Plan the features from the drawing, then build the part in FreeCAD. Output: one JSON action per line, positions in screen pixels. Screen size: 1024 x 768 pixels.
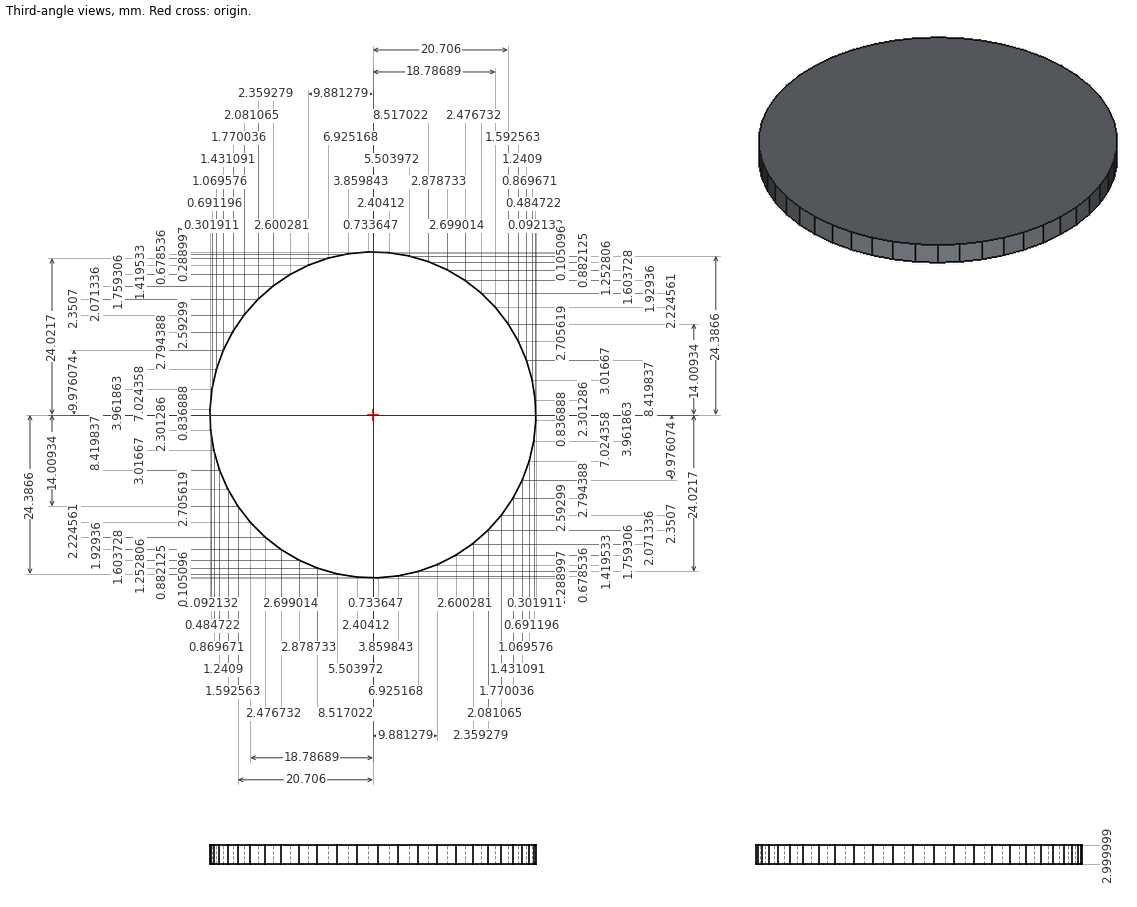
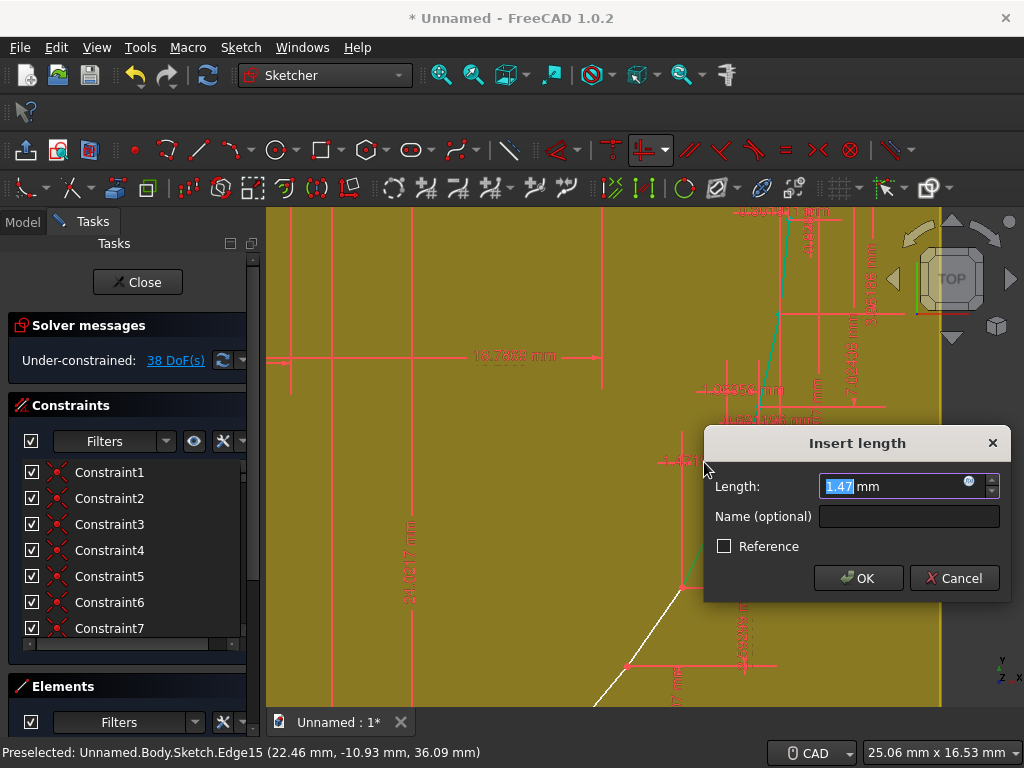
{"action": "type", "text": "1.431091"}
{"action": "key", "text": "Return"}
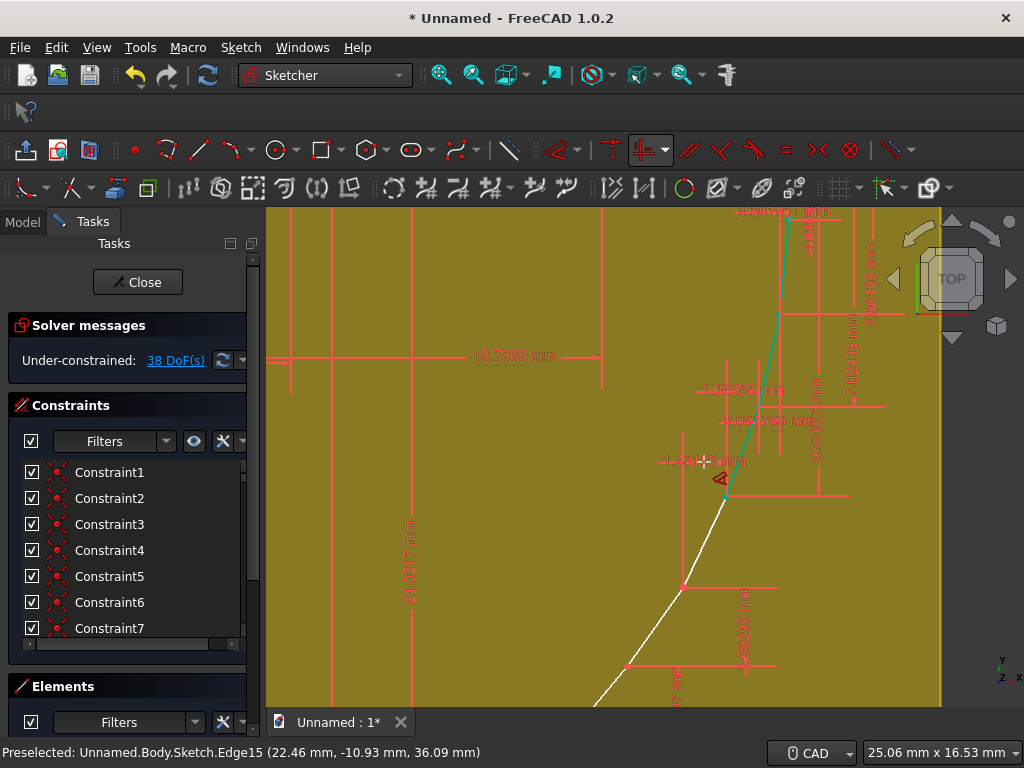
{"action": "left_click", "coordinate": [714, 524]}
{"action": "left_click", "coordinate": [761, 542]}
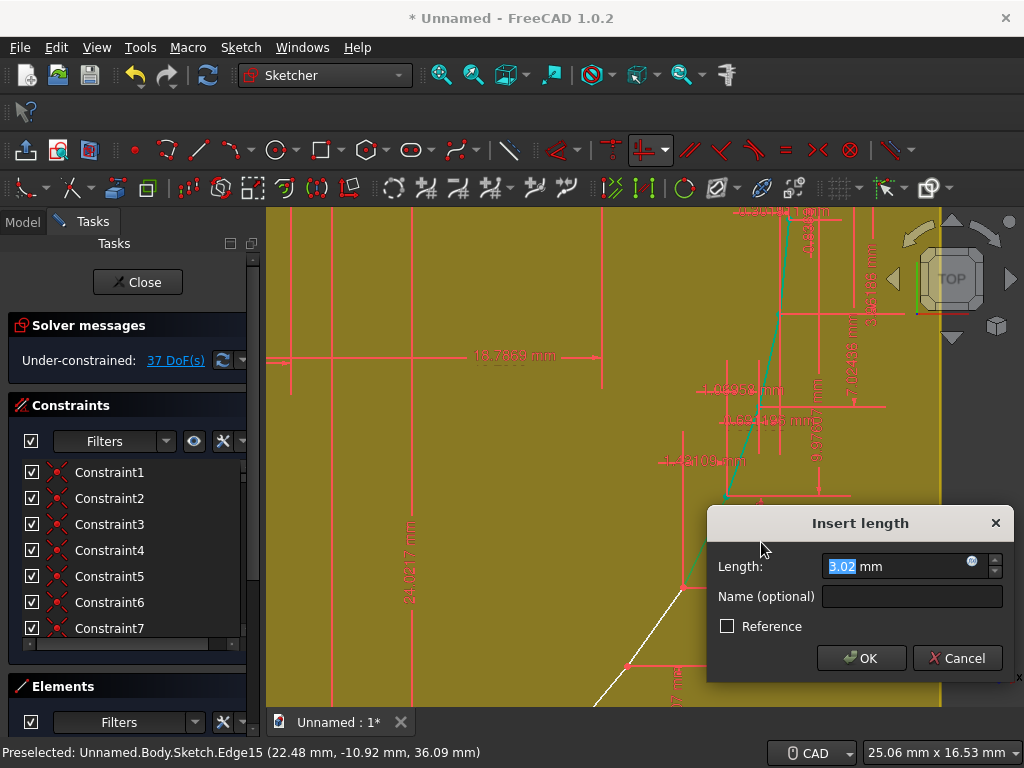
{"action": "type", "text": "2.794388"}
{"action": "key", "text": "Return"}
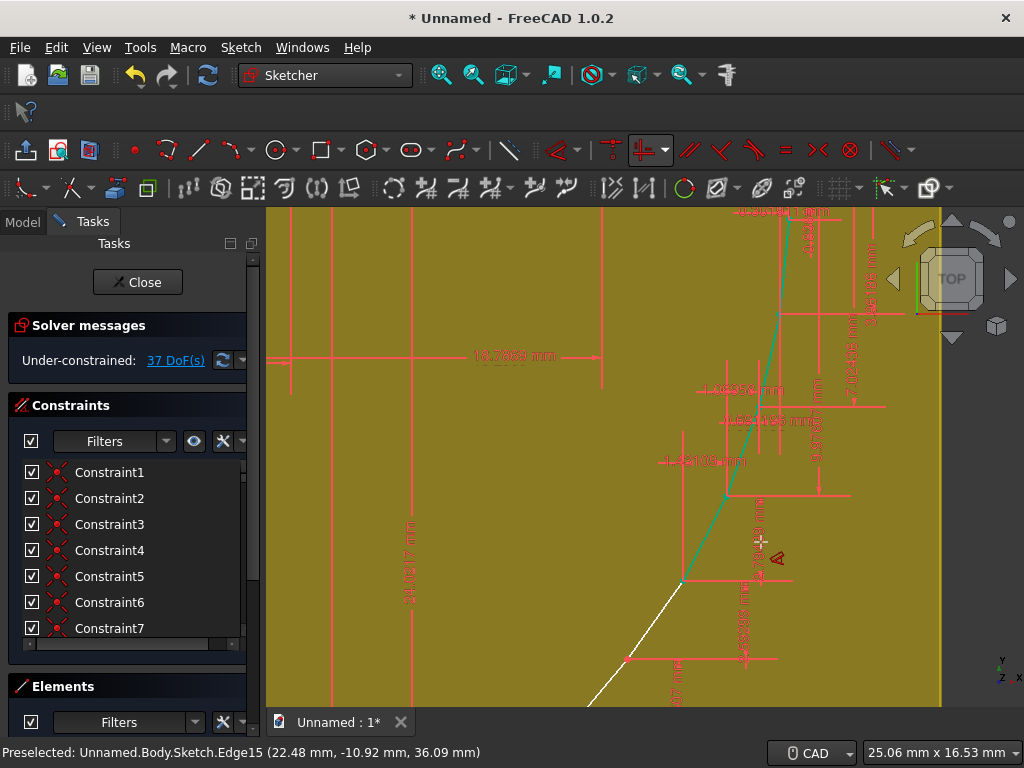
{"action": "left_click", "coordinate": [667, 604]}
{"action": "left_click", "coordinate": [656, 547]}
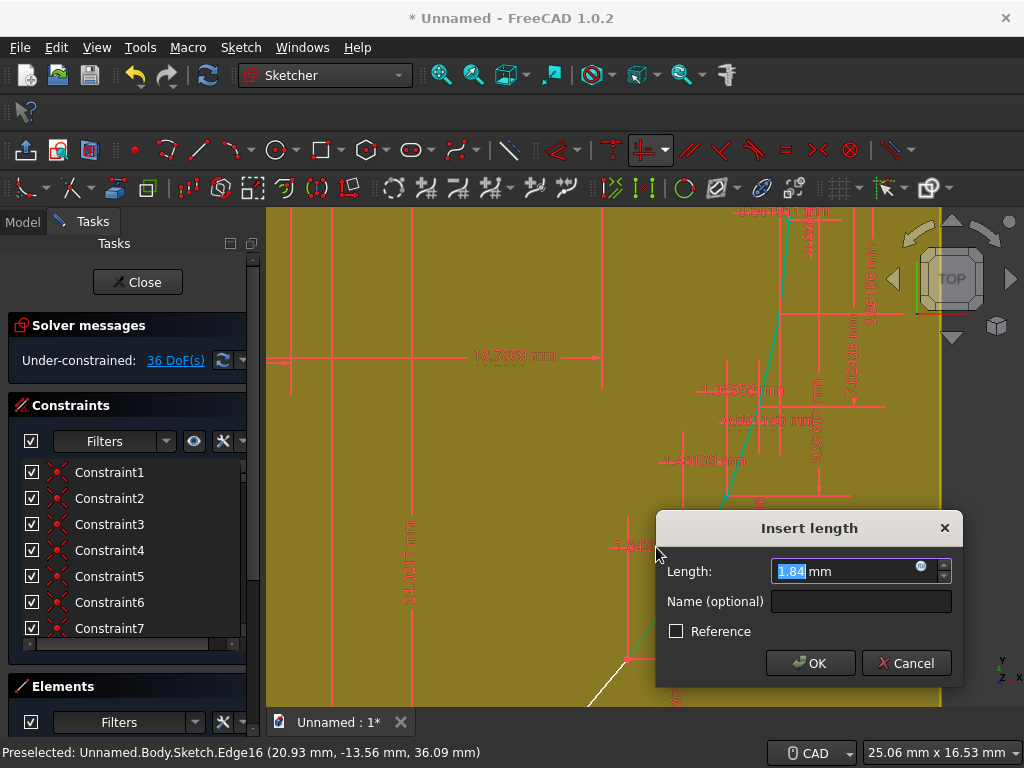
{"action": "type", "text": "1.770036"}
{"action": "key", "text": "Return"}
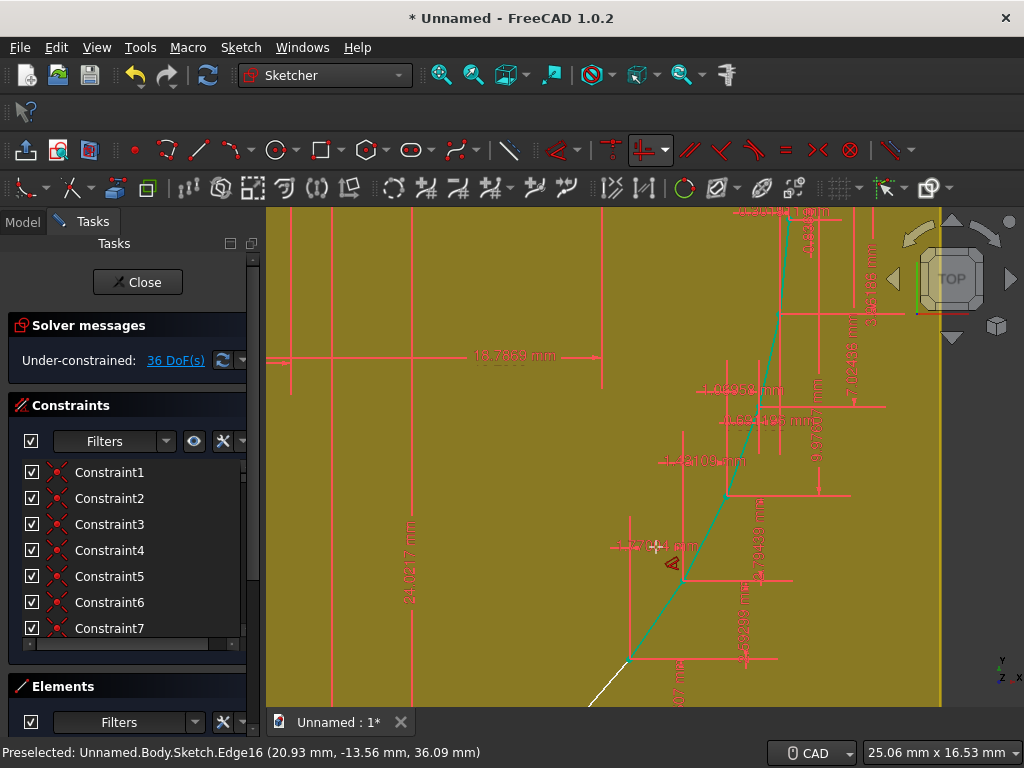
{"action": "left_click", "coordinate": [618, 673]}
{"action": "left_click", "coordinate": [599, 625]}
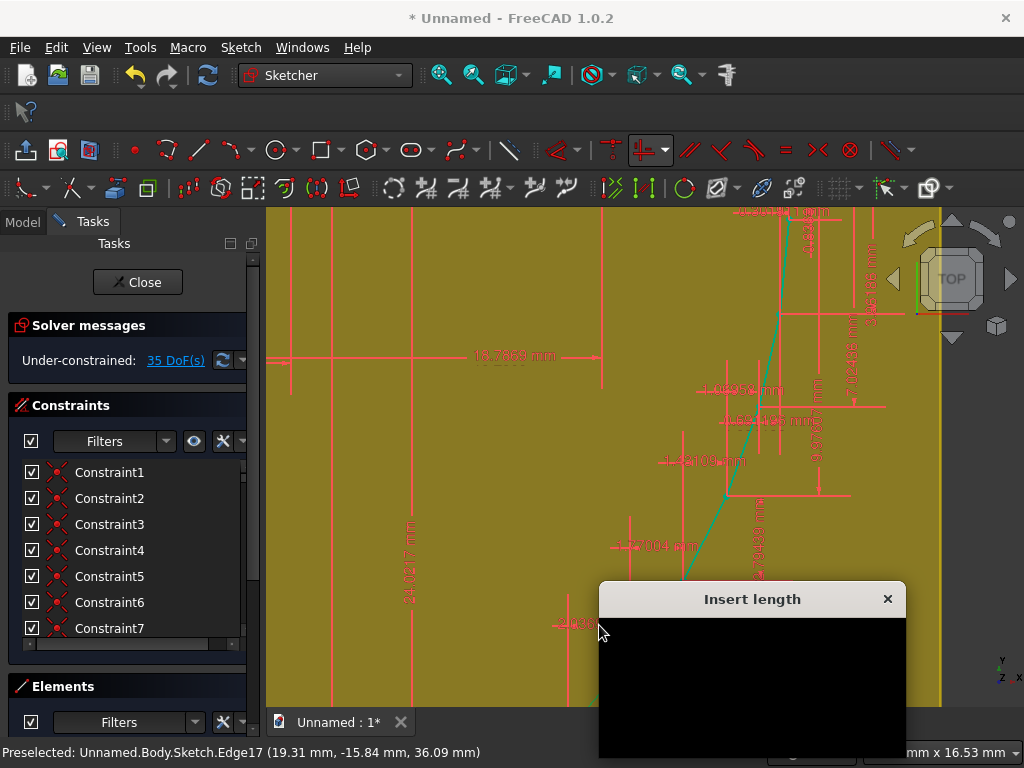
{"action": "type", "text": "2.081065"}
{"action": "key", "text": "Return"}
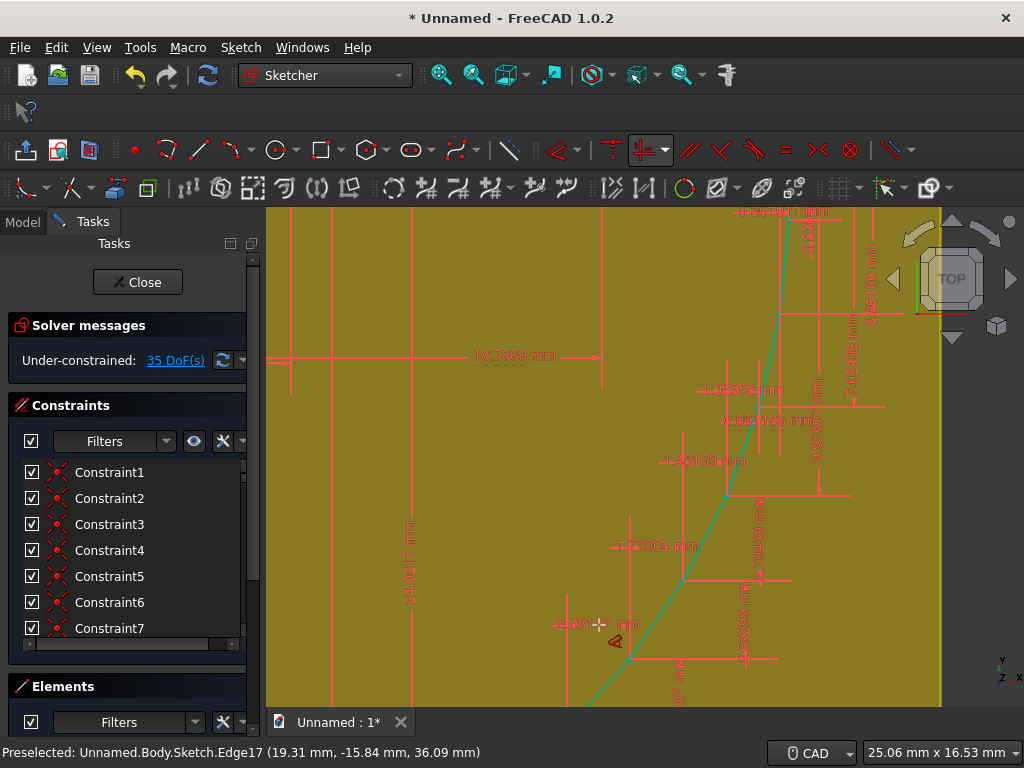
{"action": "scroll", "coordinate": [714, 523], "scroll_direction": "down", "scroll_amount": 8}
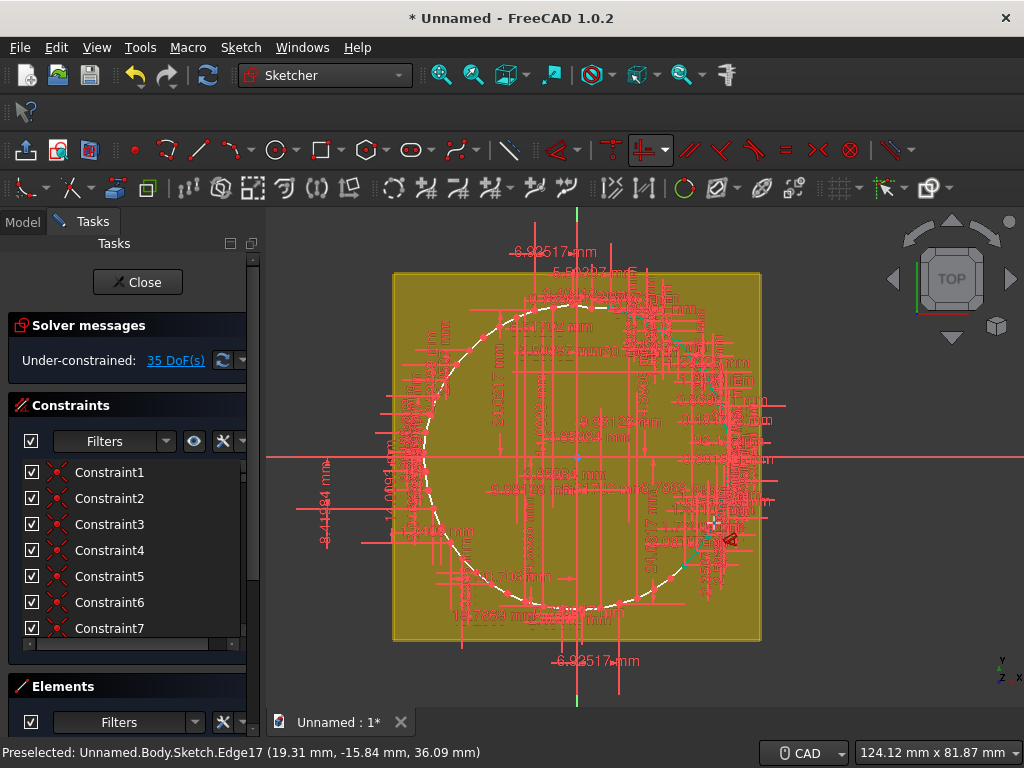
{"action": "scroll", "coordinate": [680, 569], "scroll_direction": "up", "scroll_amount": 6}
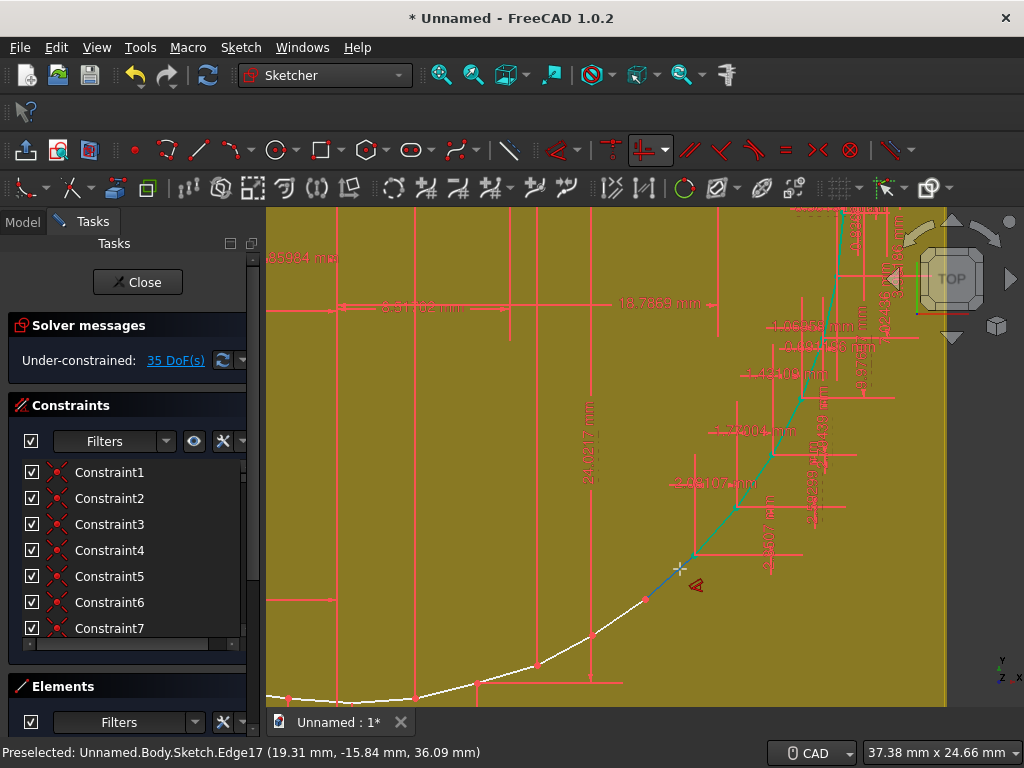
{"action": "left_click", "coordinate": [680, 568]}
{"action": "left_click", "coordinate": [670, 633]}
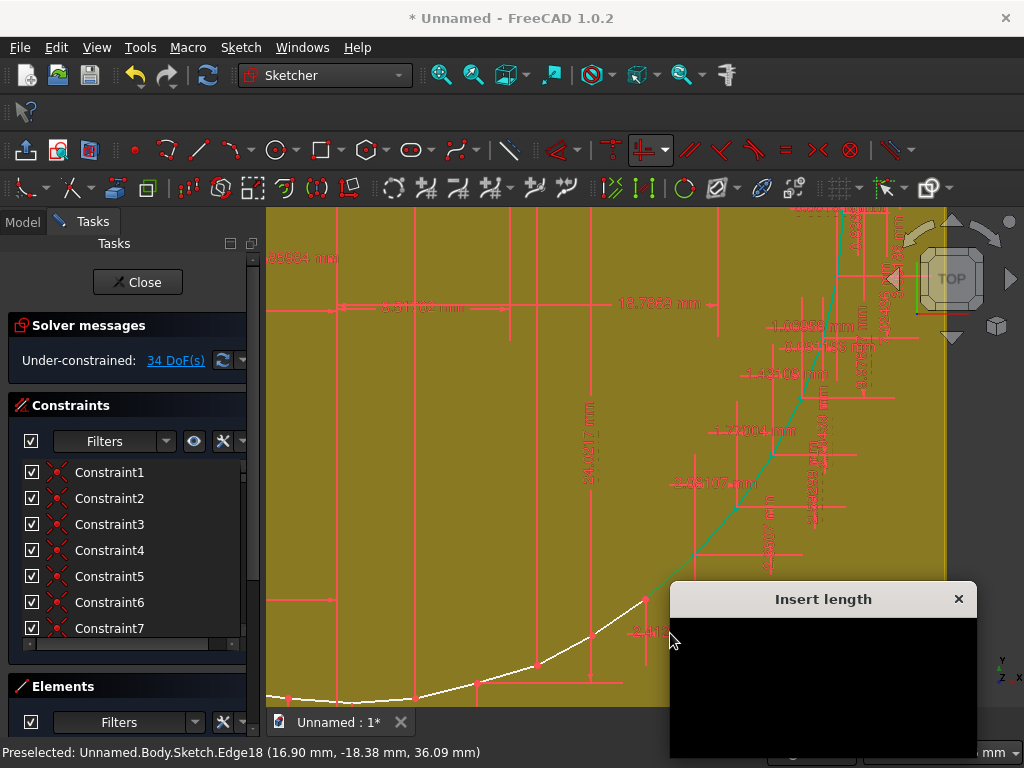
{"action": "type", "text": "2.359279"}
{"action": "key", "text": "Return"}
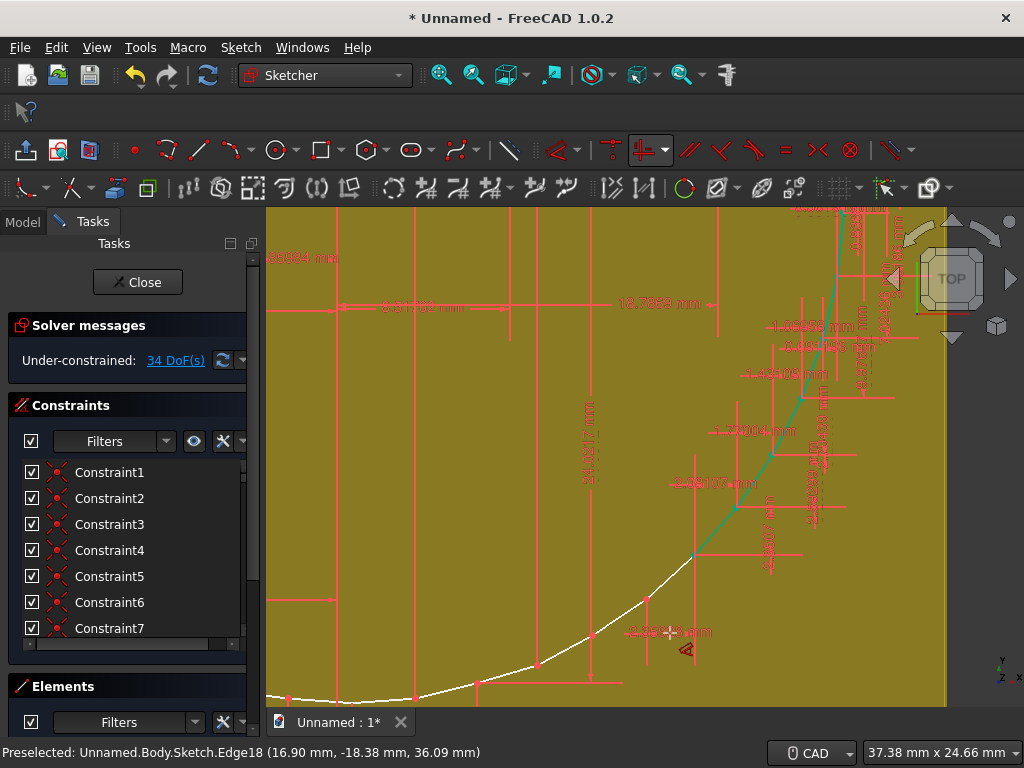
{"action": "left_click", "coordinate": [680, 568]}
{"action": "left_click", "coordinate": [729, 577]}